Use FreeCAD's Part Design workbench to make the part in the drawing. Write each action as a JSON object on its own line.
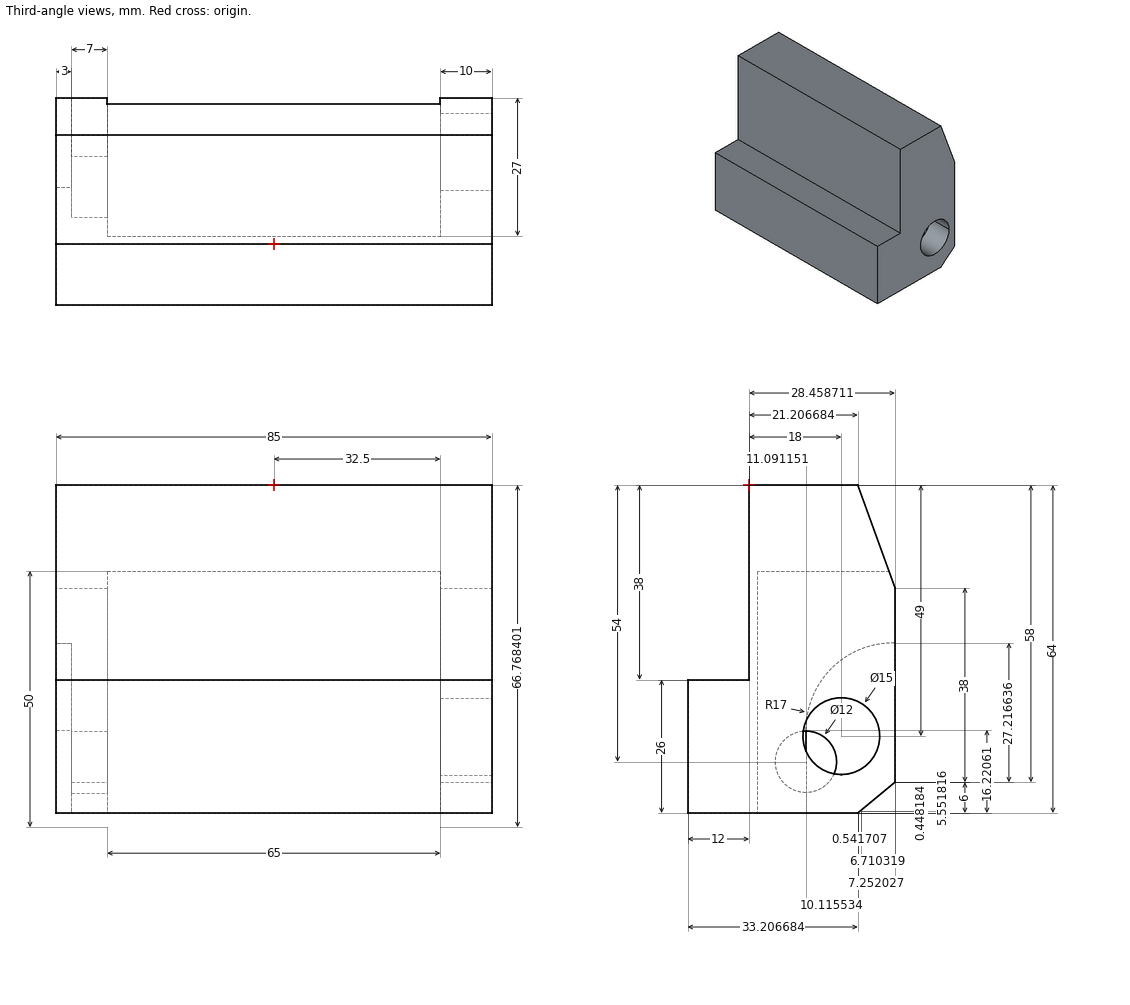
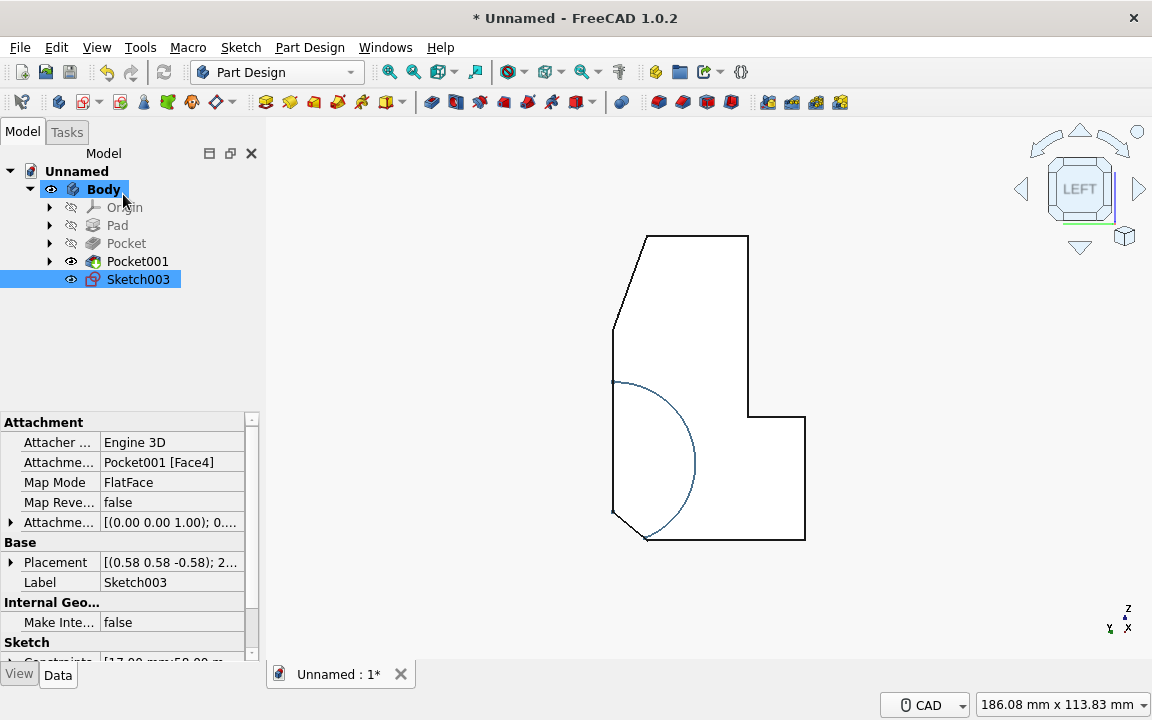
{"action": "left_click", "coordinate": [432, 102]}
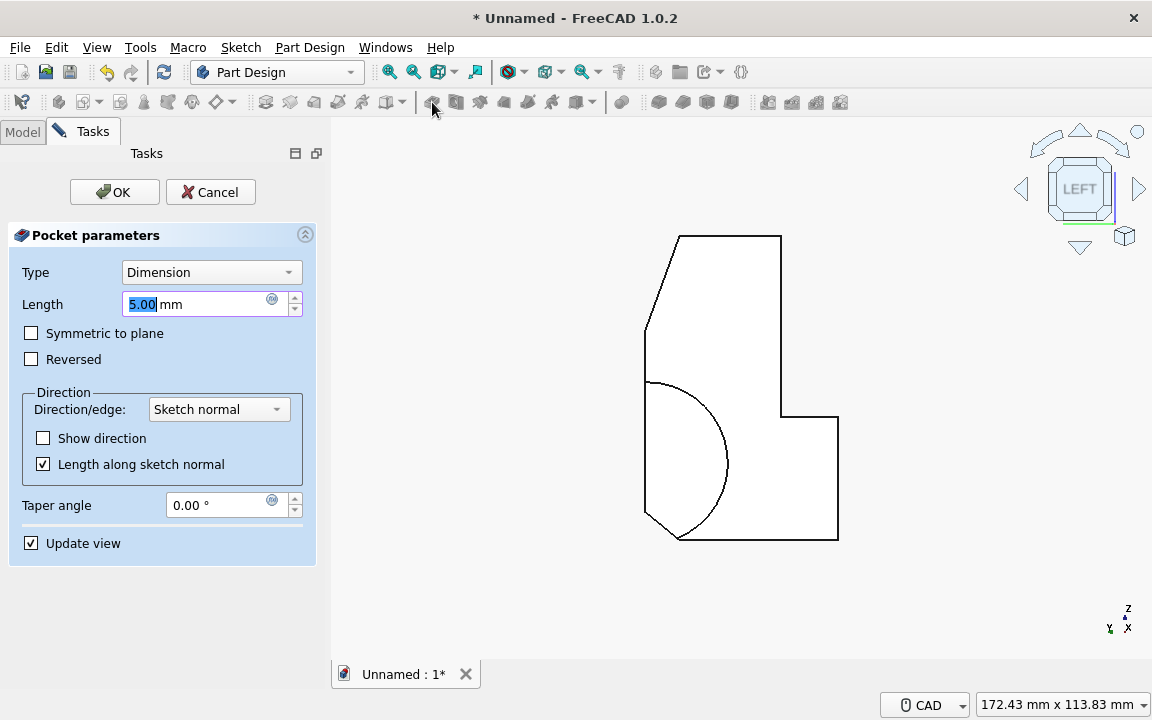
{"action": "type", "text": "3"}
{"action": "key", "text": "Tab"}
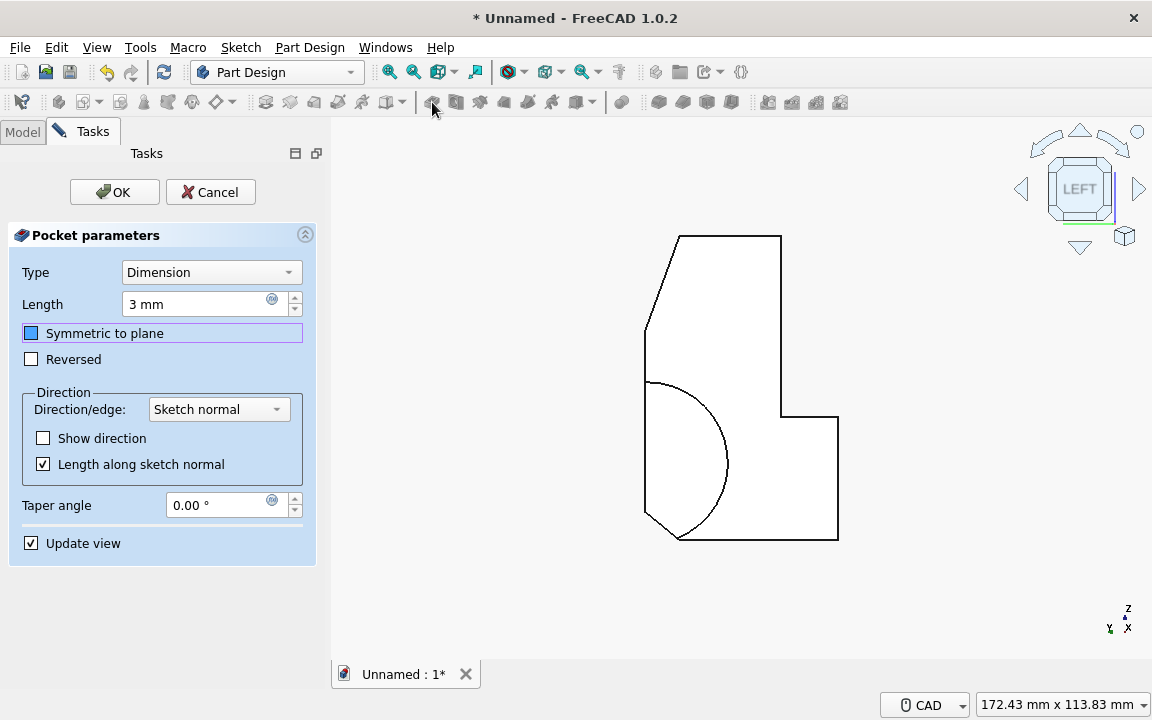
{"action": "left_click", "coordinate": [115, 192]}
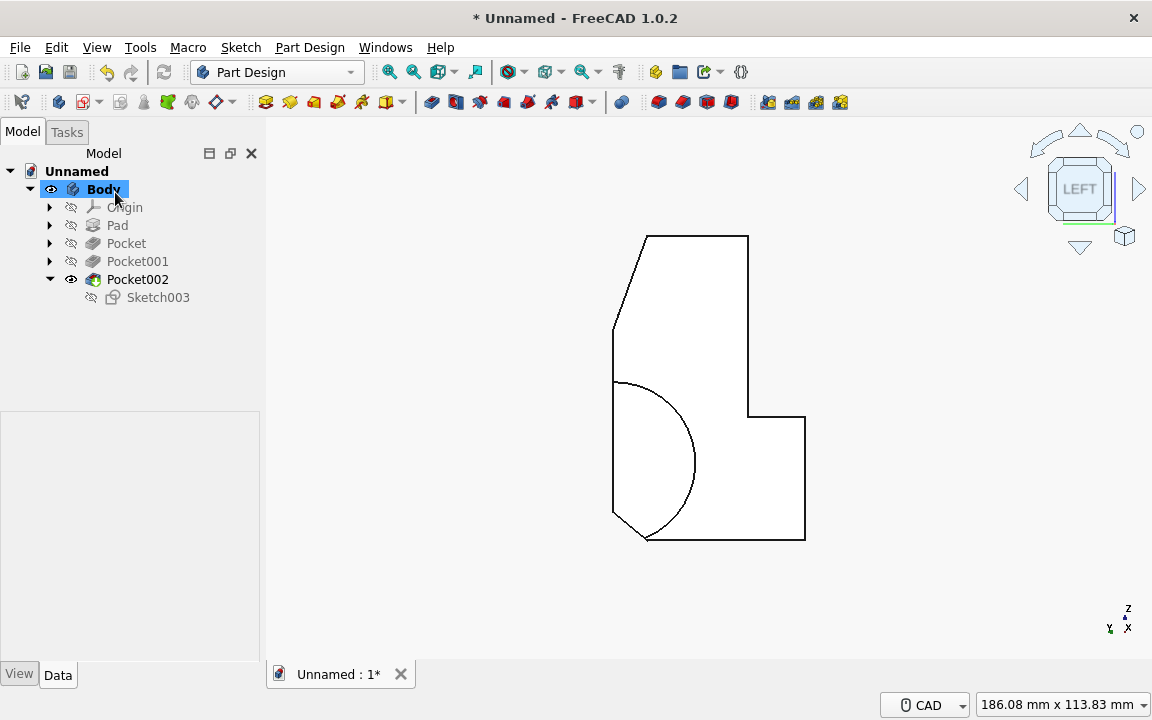
{"action": "left_click", "coordinate": [681, 343]}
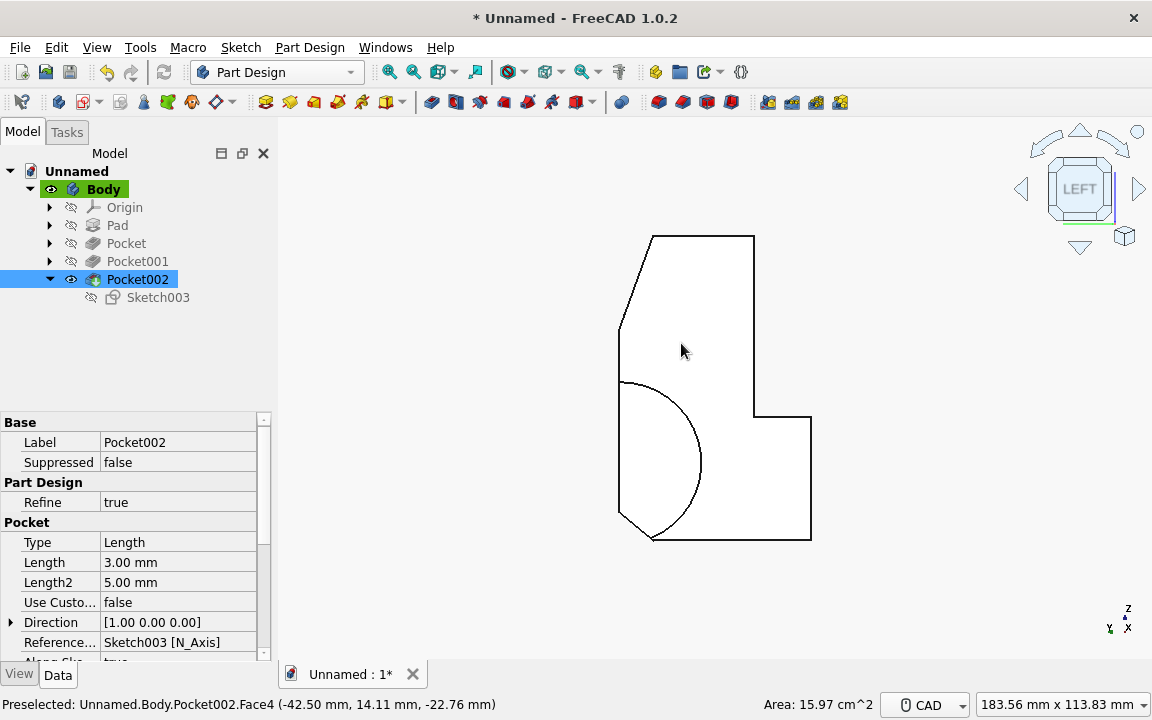
{"action": "left_click", "coordinate": [84, 102]}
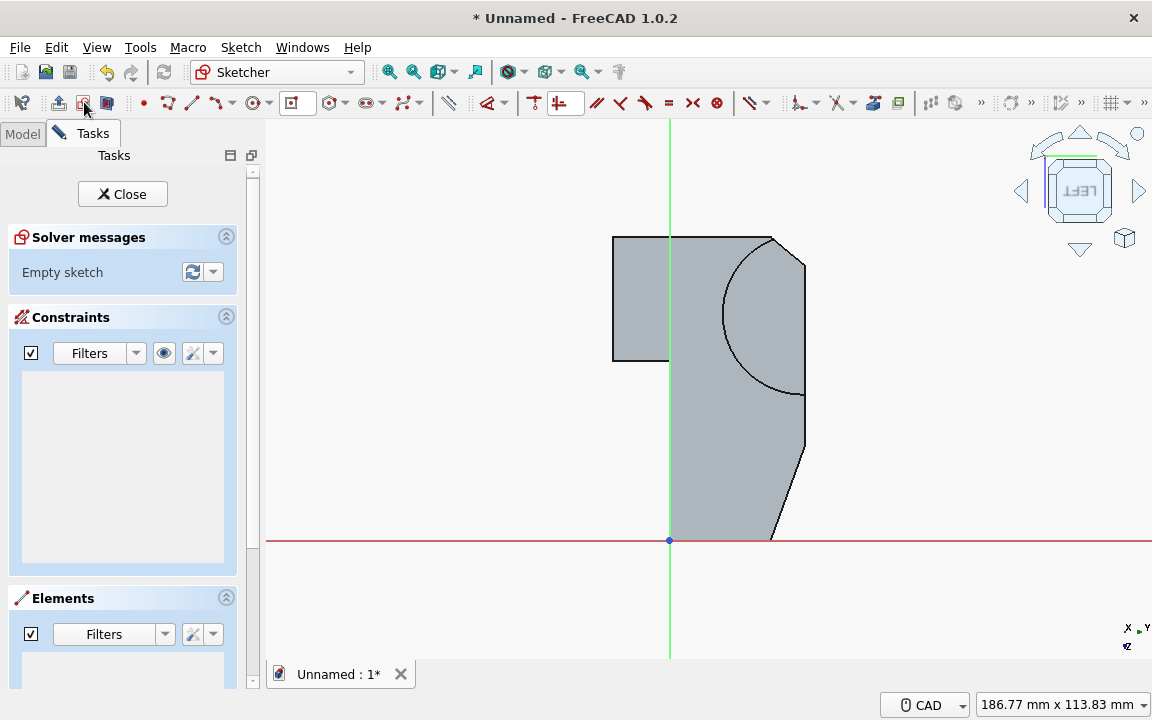
{"action": "scroll", "coordinate": [783, 239], "scroll_direction": "up", "scroll_amount": 7}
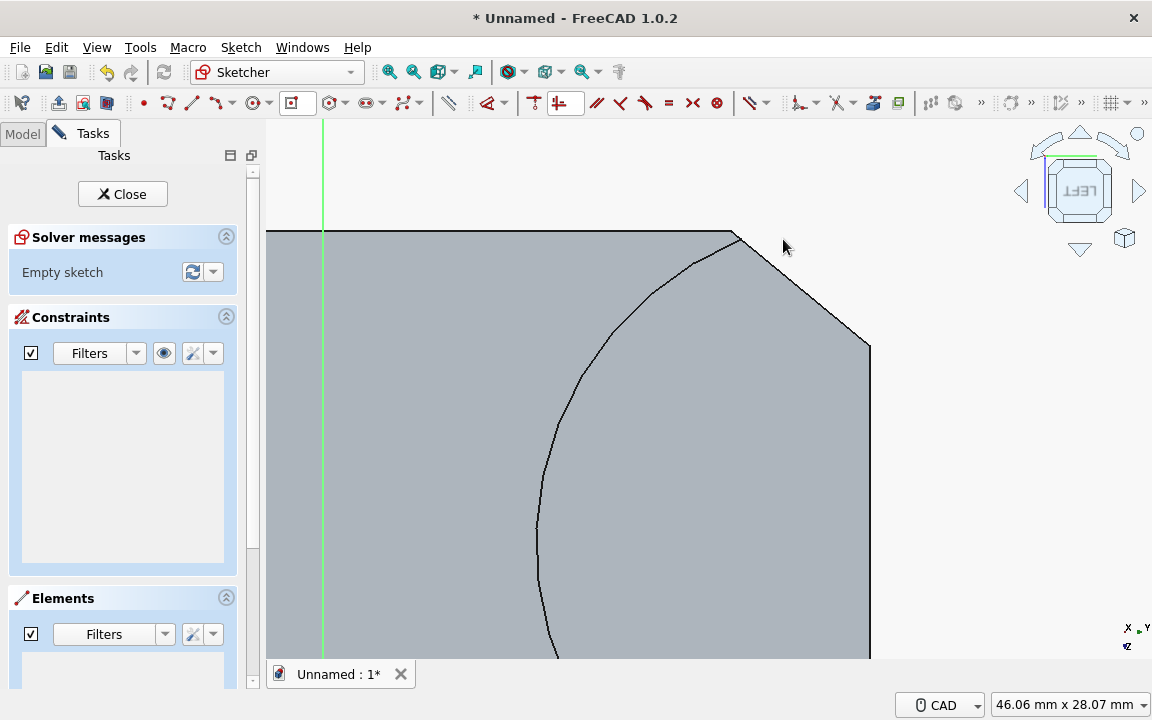
{"action": "left_click", "coordinate": [168, 104]}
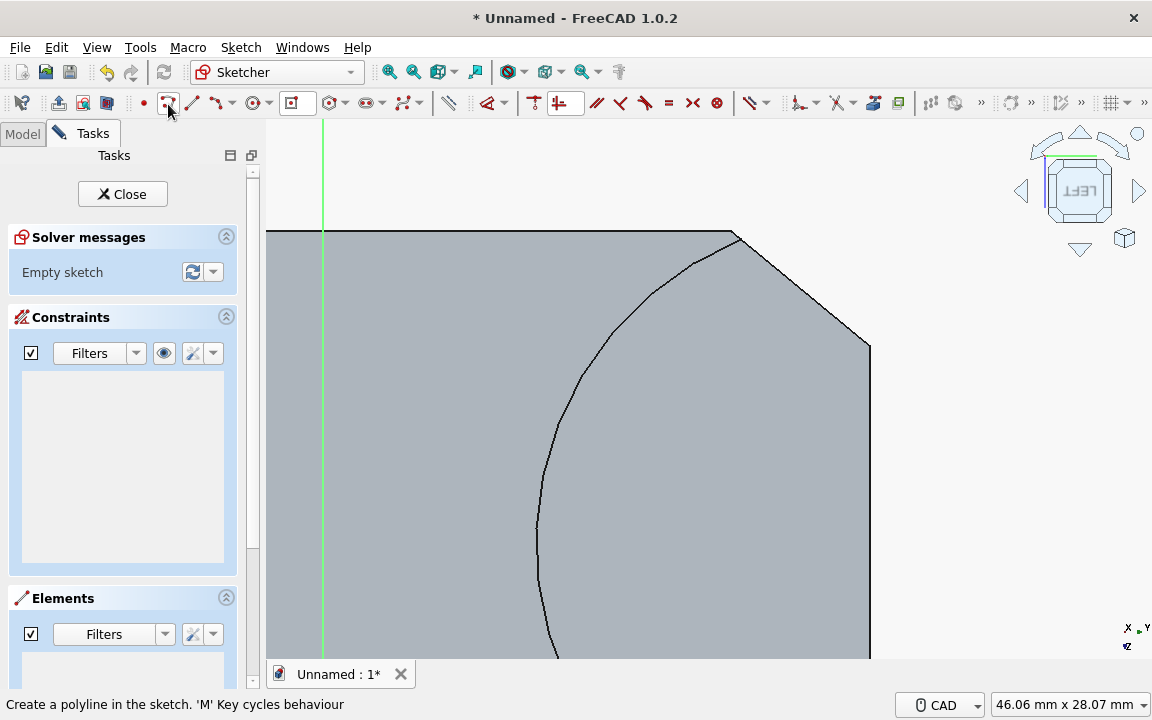
{"action": "left_click", "coordinate": [536, 543]}
{"action": "left_click", "coordinate": [741, 240]}
{"action": "left_click", "coordinate": [731, 231]}
{"action": "left_click", "coordinate": [536, 231]}
{"action": "left_click", "coordinate": [536, 544]}
{"action": "key", "text": "Escape"}
{"action": "key", "text": "Escape"}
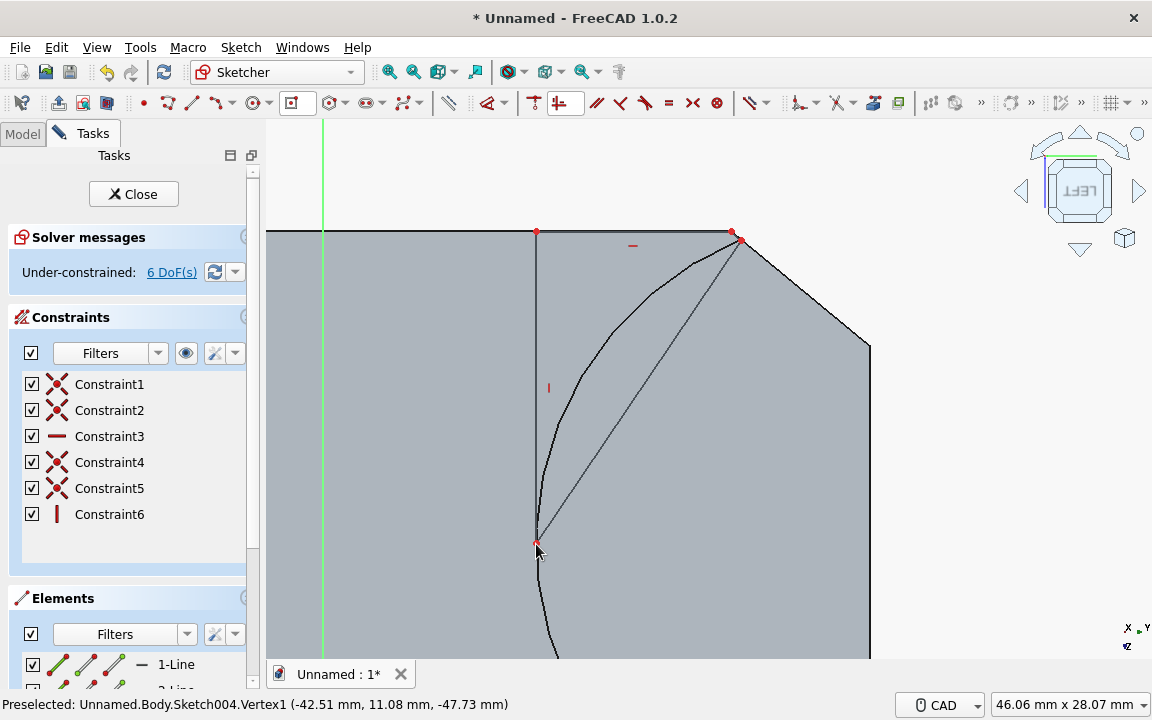
{"action": "left_click", "coordinate": [488, 104]}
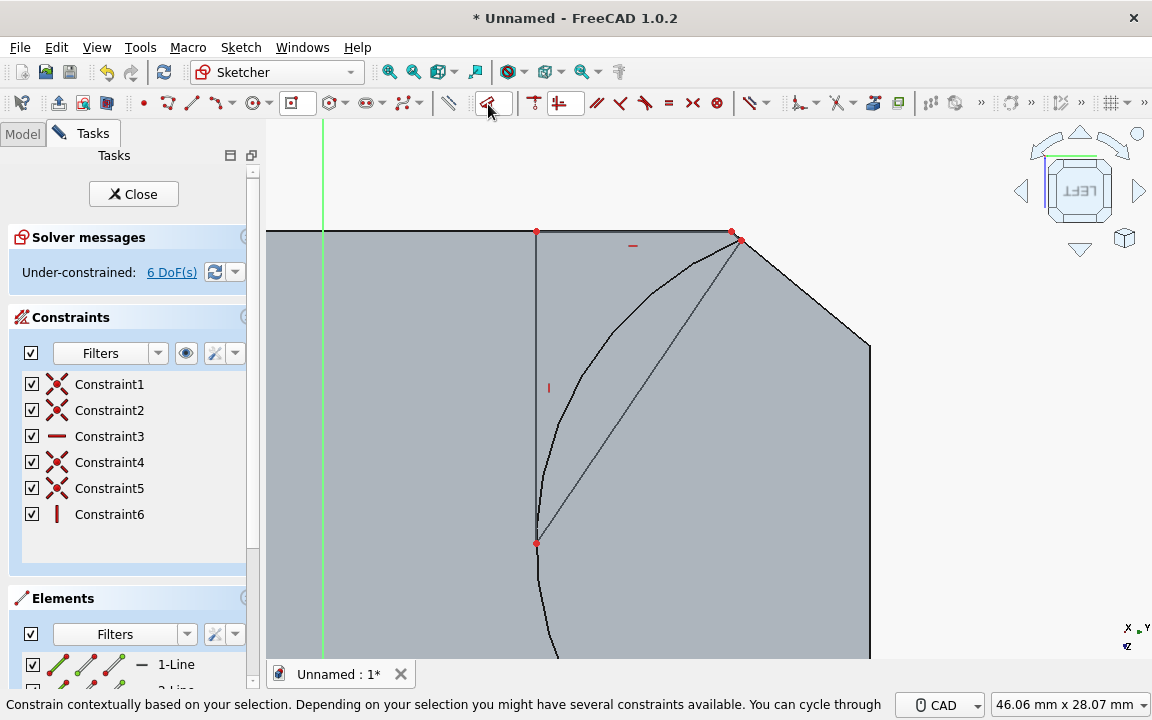
{"action": "left_click", "coordinate": [731, 232]}
{"action": "left_click", "coordinate": [765, 432]}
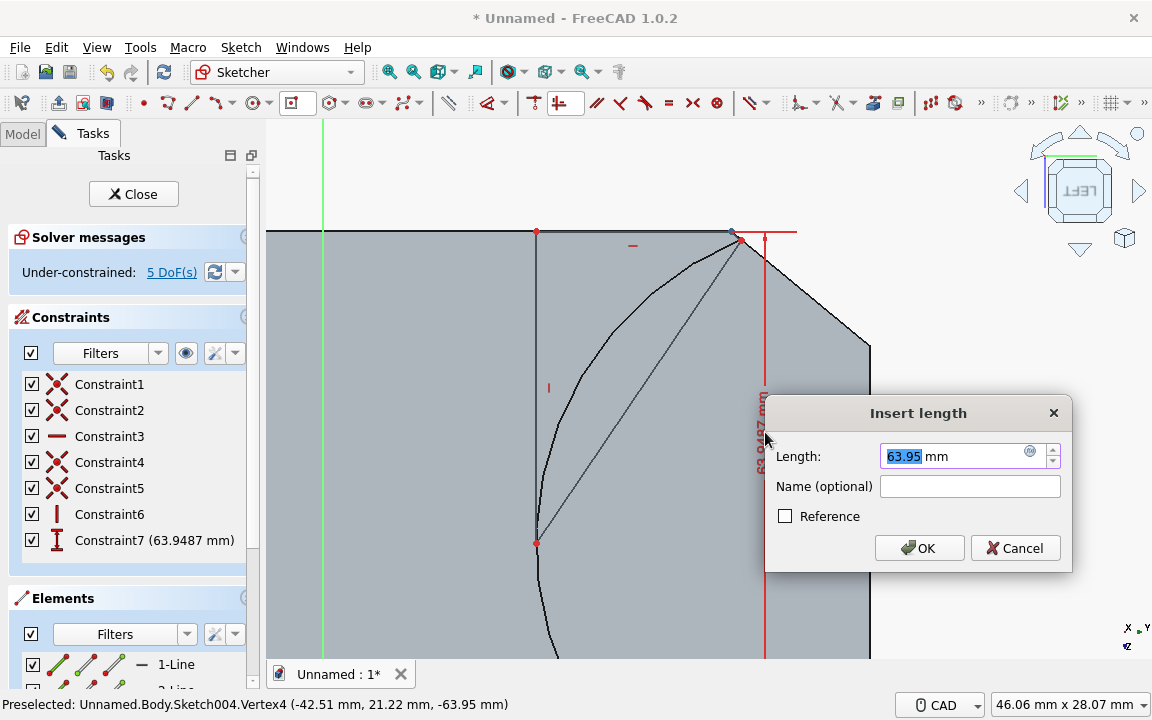
{"action": "type", "text": "64"}
{"action": "key", "text": "Return"}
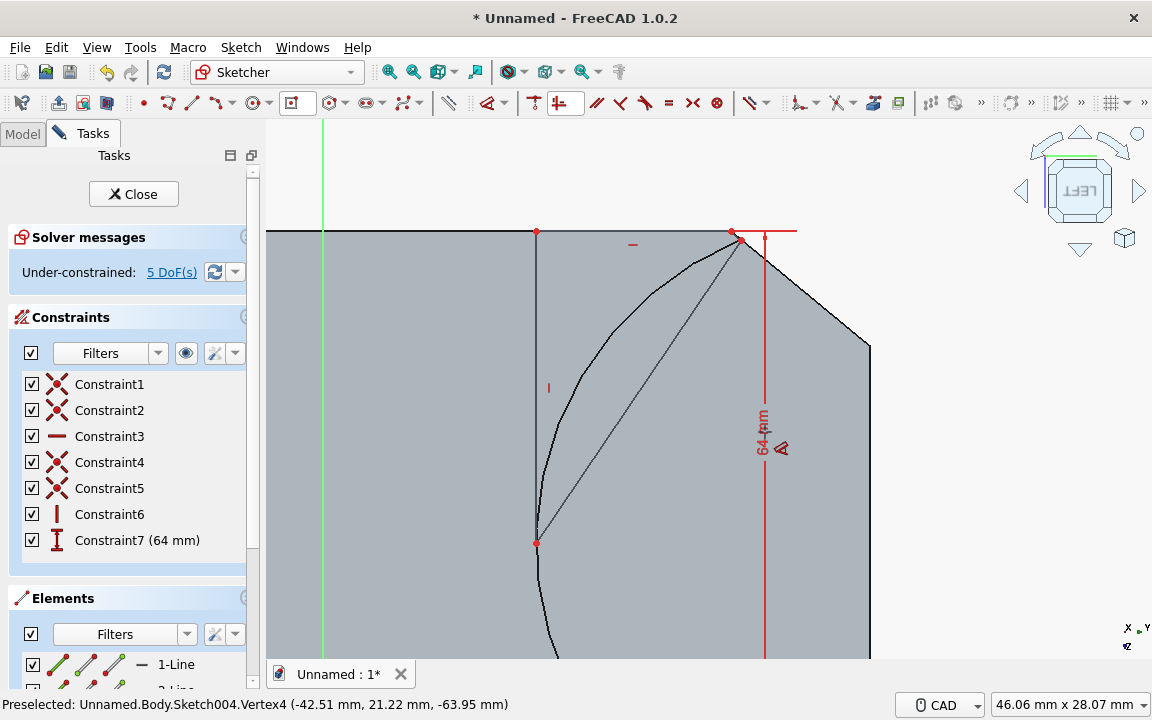
{"action": "left_click", "coordinate": [536, 325]}
{"action": "left_click", "coordinate": [502, 388]}